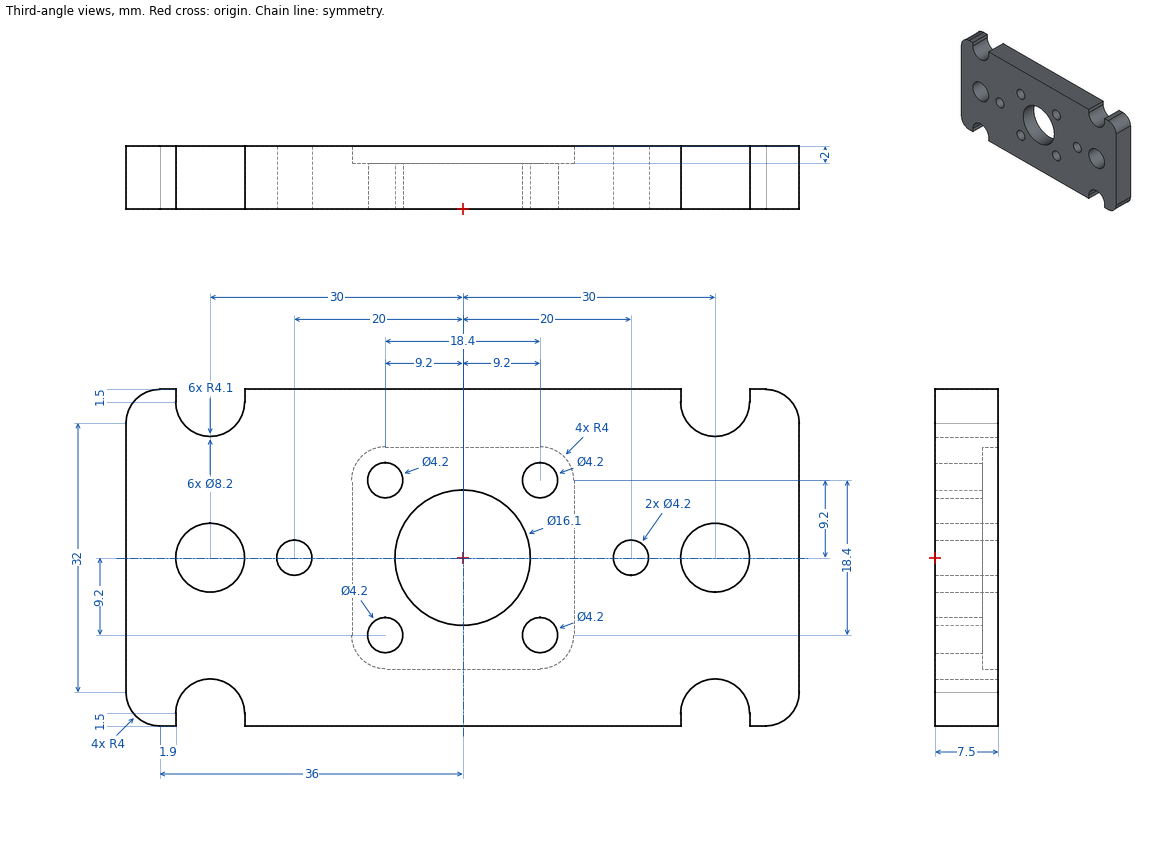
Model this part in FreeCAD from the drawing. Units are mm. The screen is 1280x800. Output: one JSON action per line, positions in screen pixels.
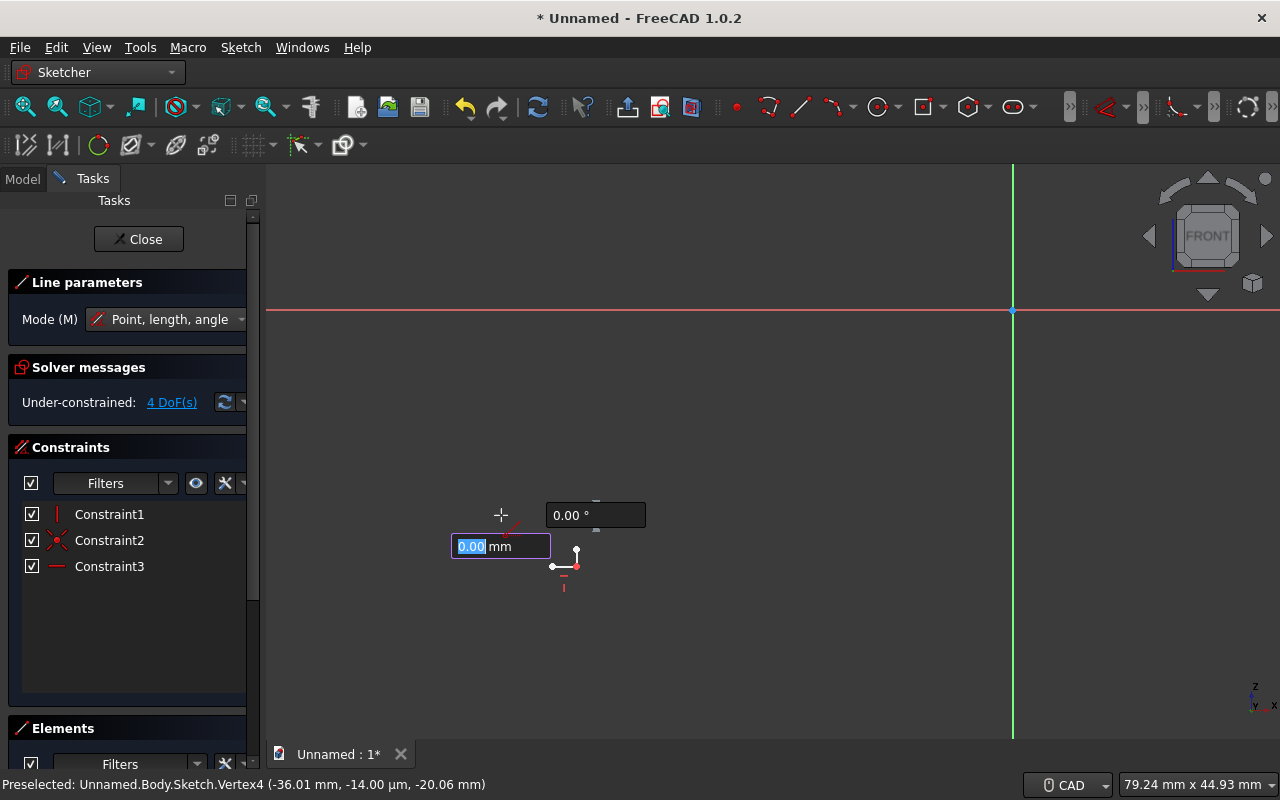
{"action": "scroll", "coordinate": [329, 623], "scroll_direction": "down", "scroll_amount": 3}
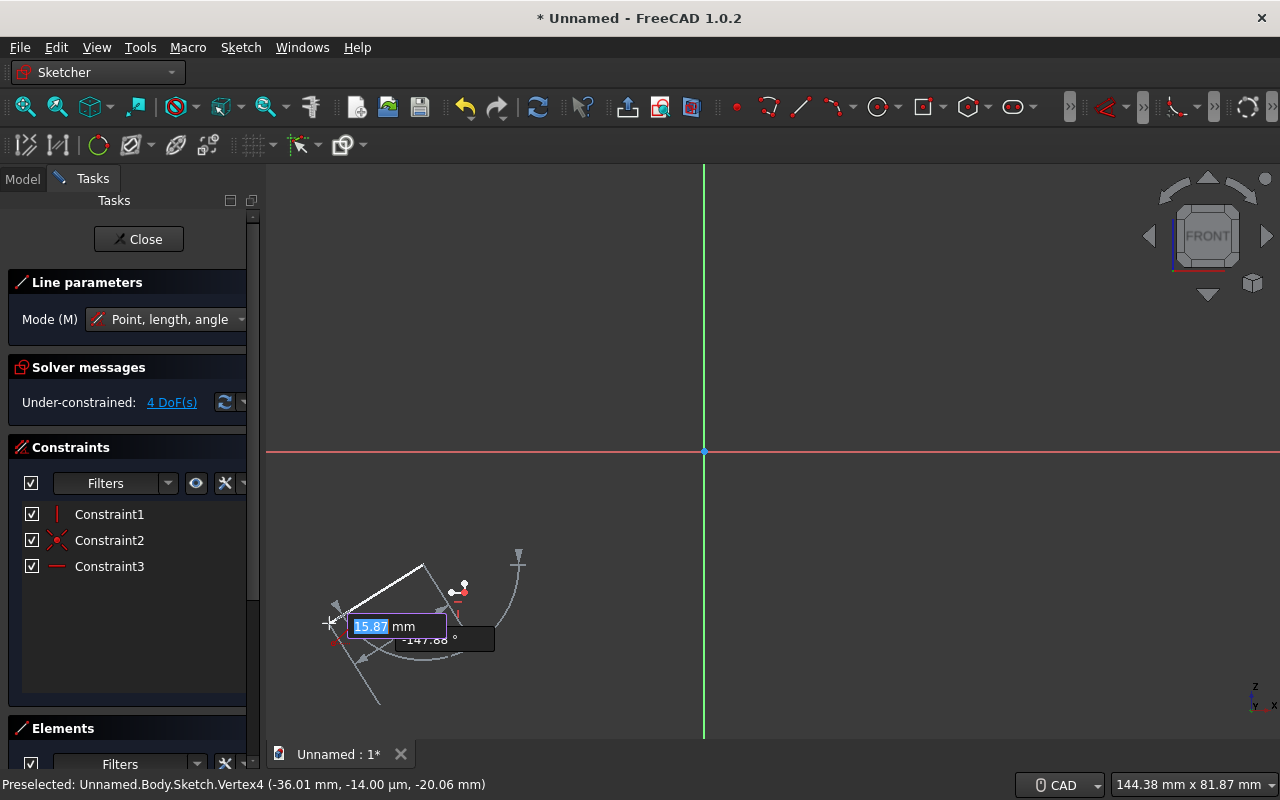
{"action": "left_click", "coordinate": [423, 339]}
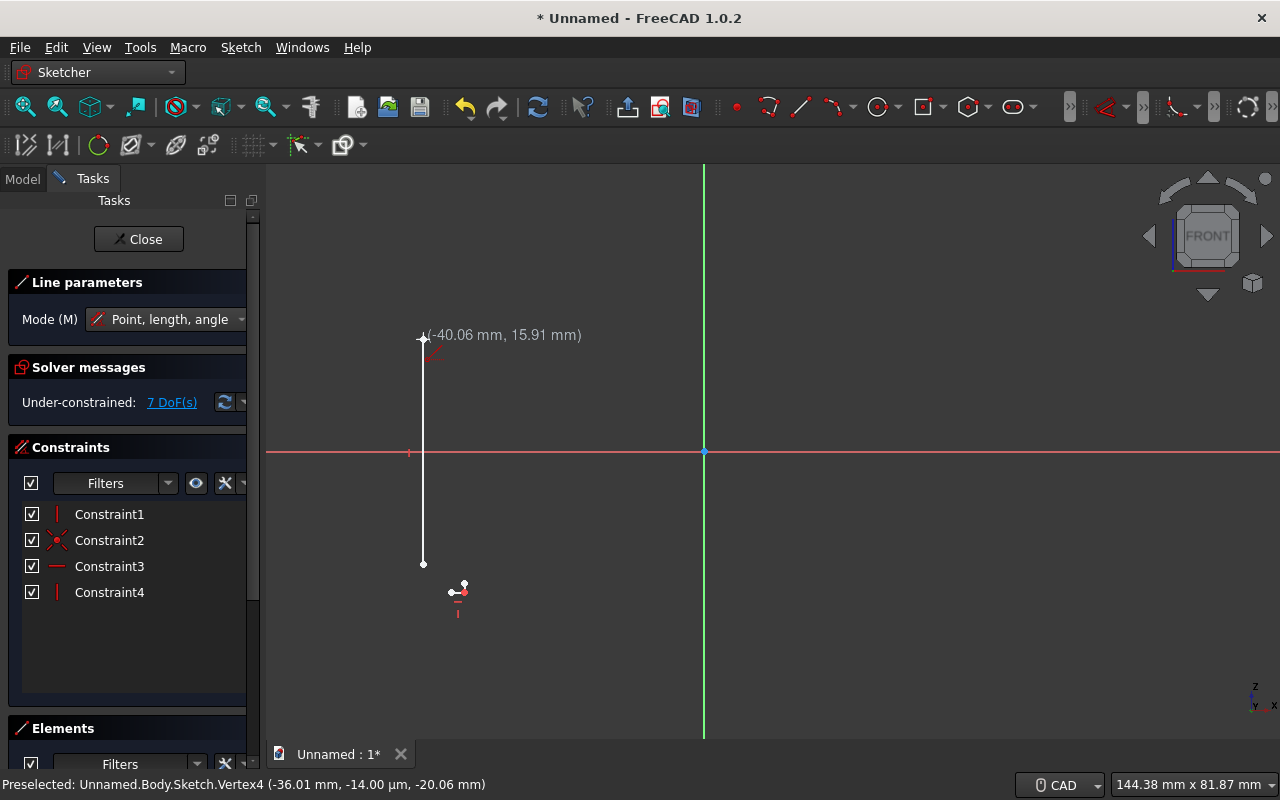
{"action": "left_click", "coordinate": [770, 108]}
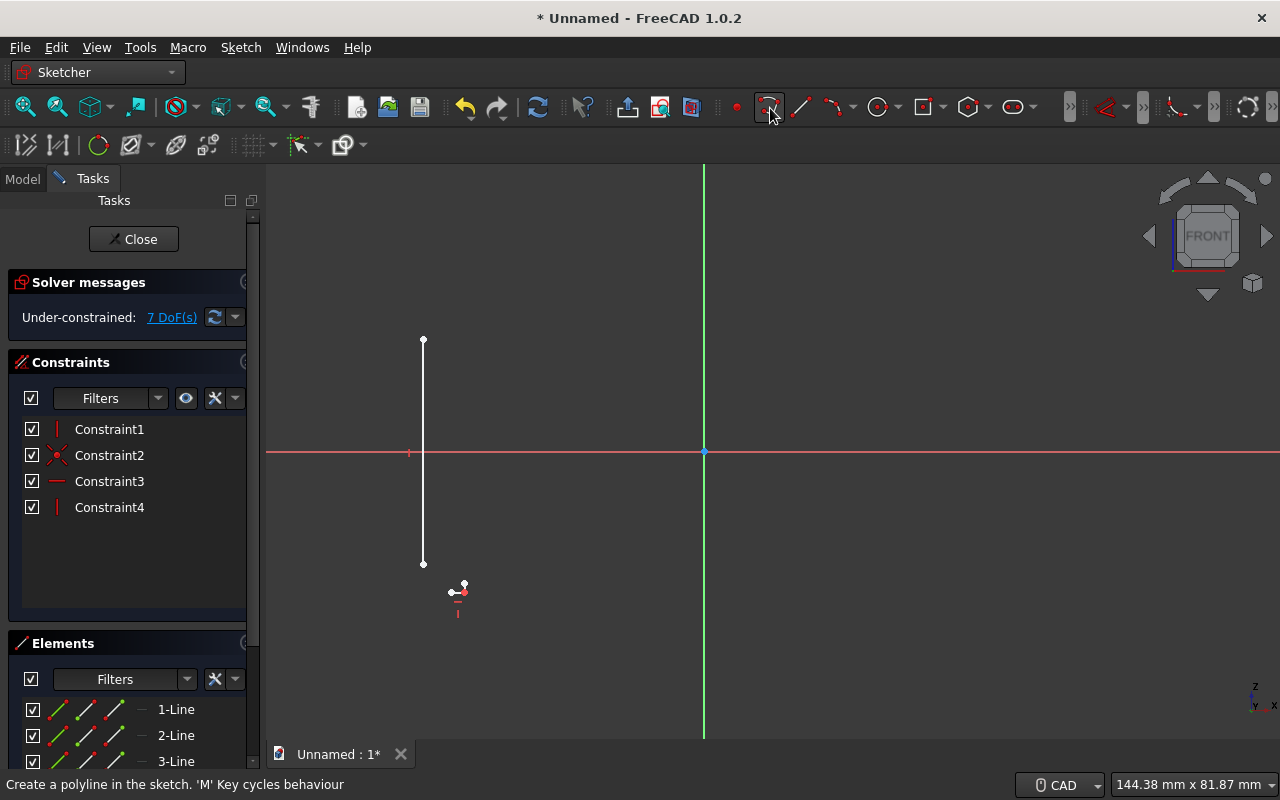
{"action": "left_click", "coordinate": [451, 311]}
{"action": "left_click", "coordinate": [465, 311]}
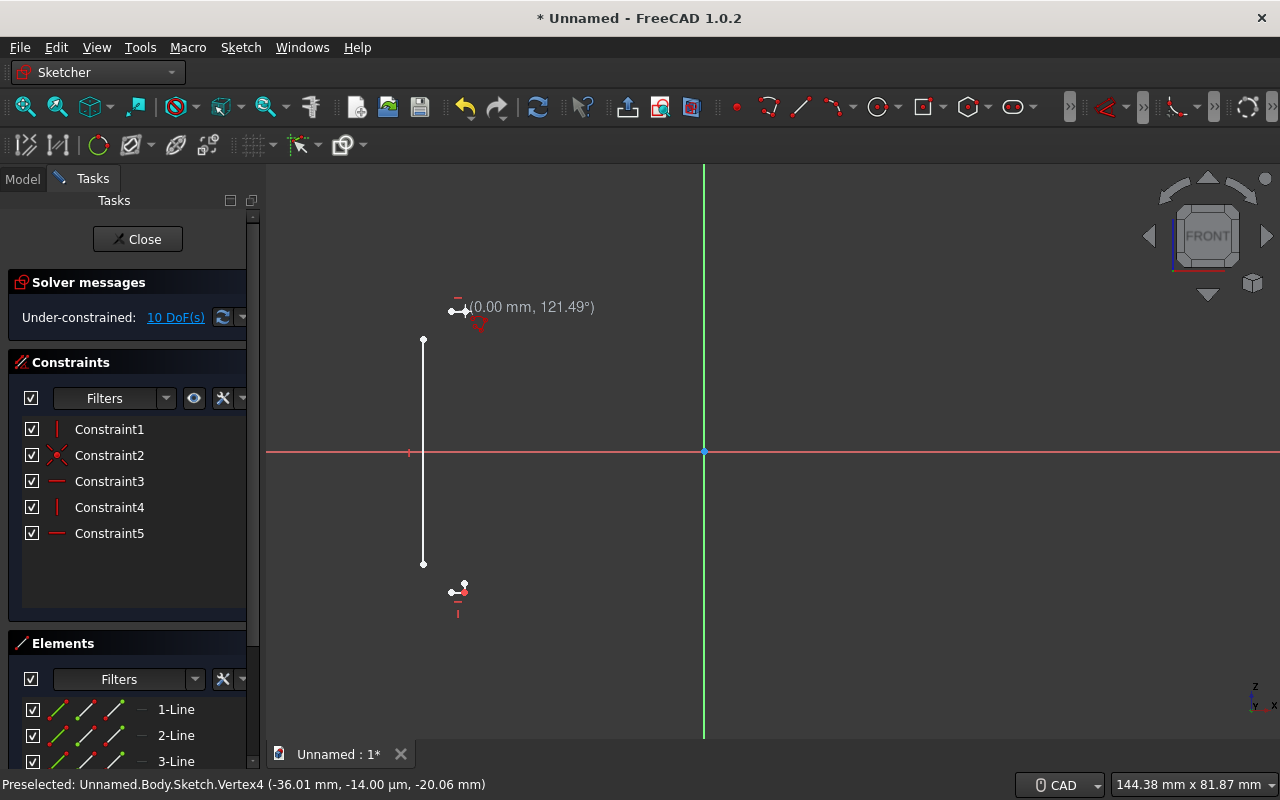
{"action": "scroll", "coordinate": [465, 322], "scroll_direction": "up", "scroll_amount": 3}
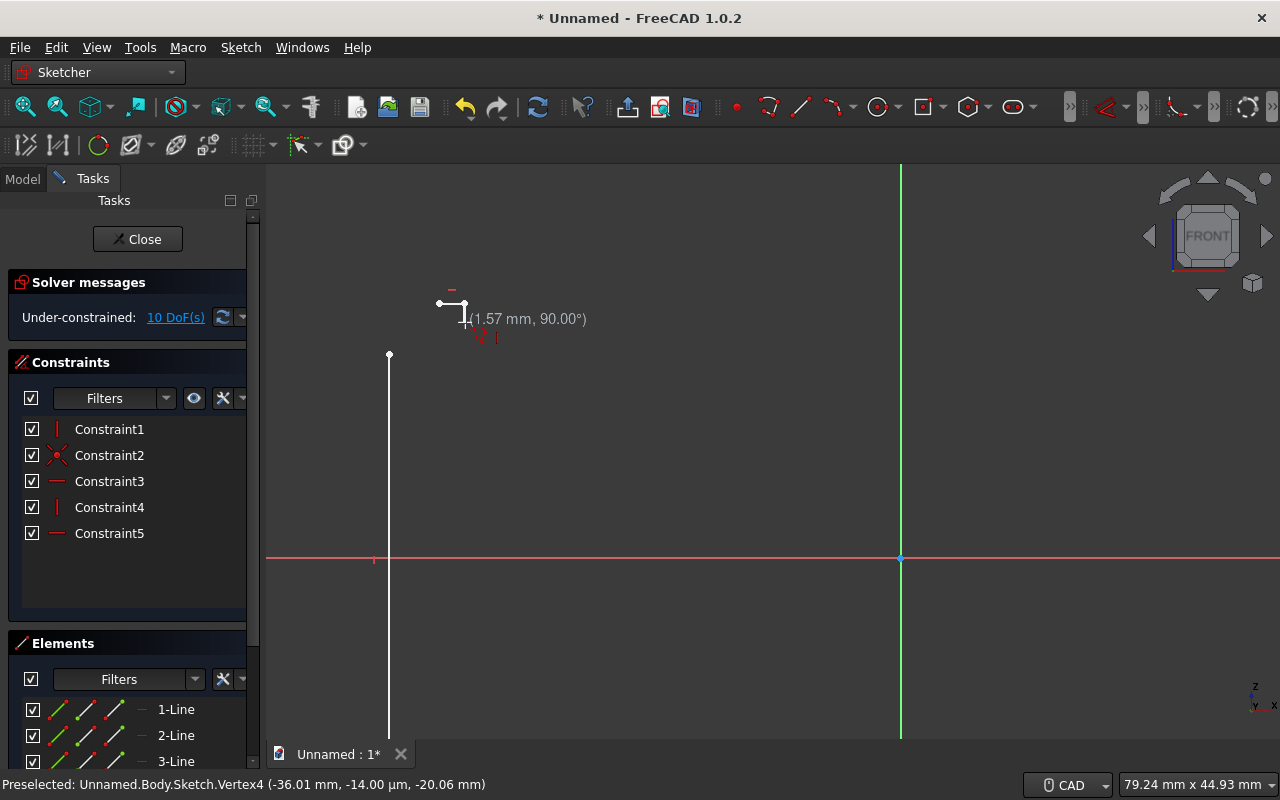
{"action": "left_click", "coordinate": [465, 321]}
{"action": "right_click", "coordinate": [465, 321]}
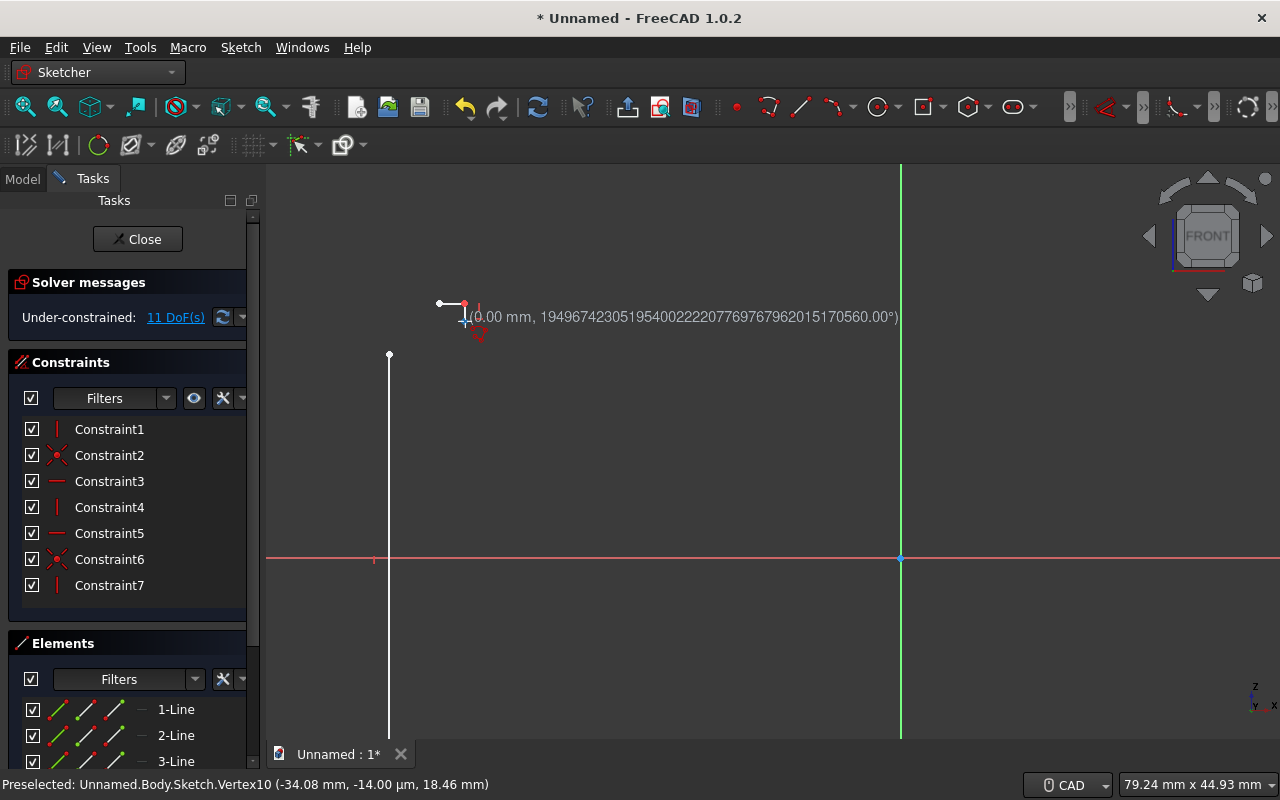
{"action": "left_click", "coordinate": [569, 321]}
{"action": "left_click", "coordinate": [569, 302]}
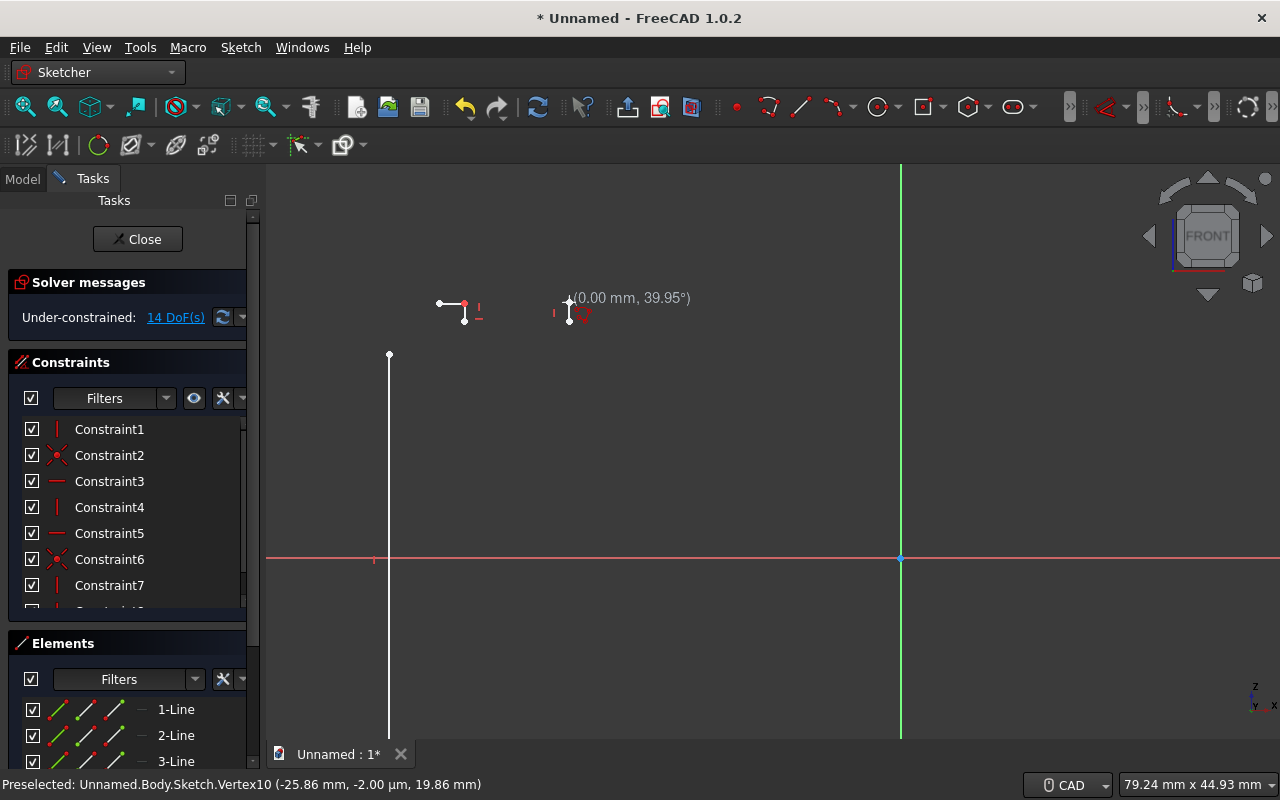
{"action": "scroll", "coordinate": [466, 322], "scroll_direction": "down", "scroll_amount": 3}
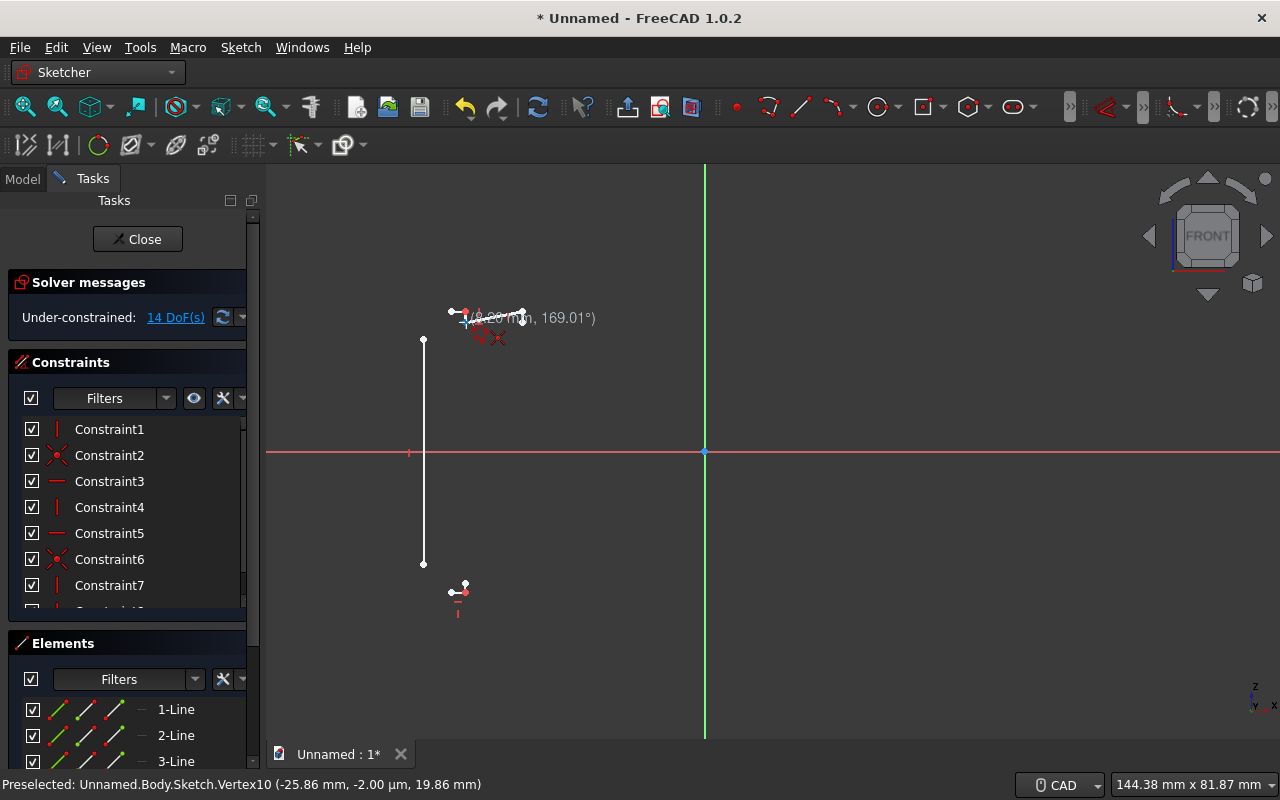
{"action": "left_click", "coordinate": [887, 311]}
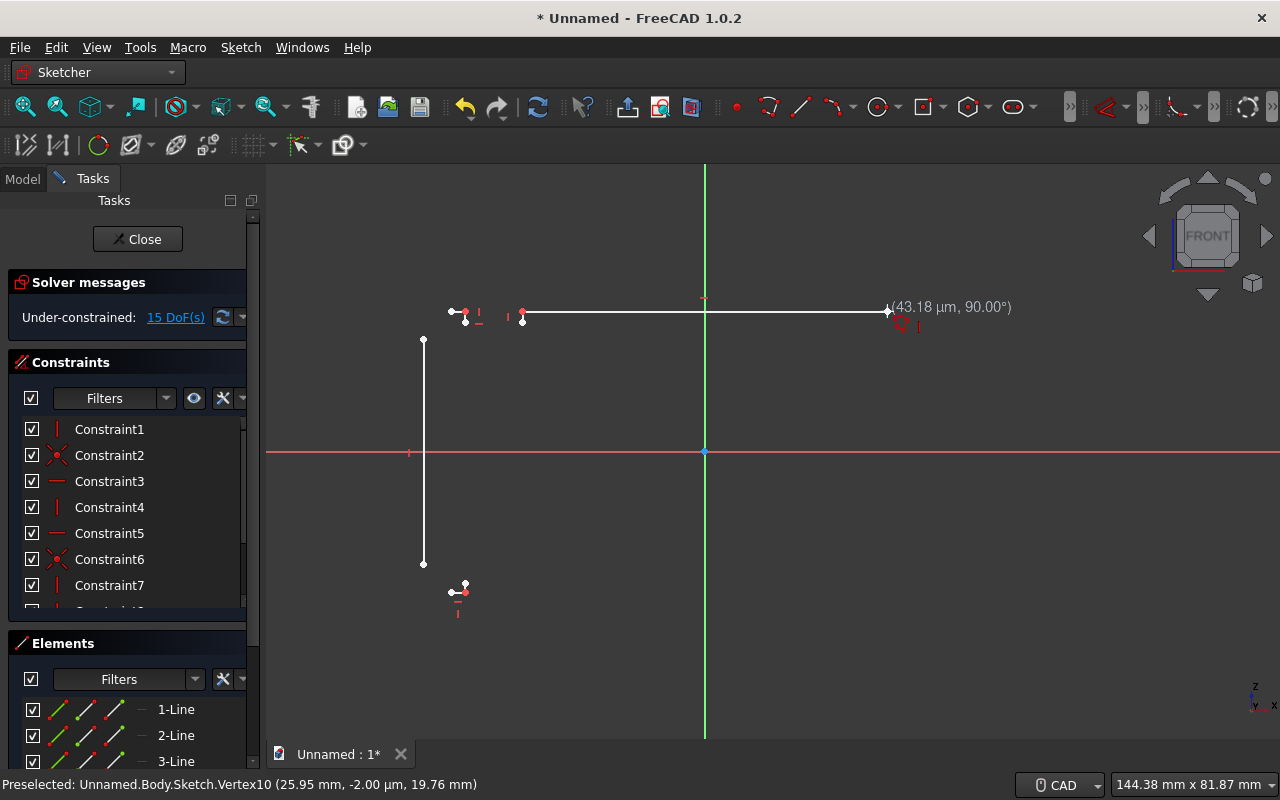
{"action": "scroll", "coordinate": [887, 322], "scroll_direction": "up", "scroll_amount": 3}